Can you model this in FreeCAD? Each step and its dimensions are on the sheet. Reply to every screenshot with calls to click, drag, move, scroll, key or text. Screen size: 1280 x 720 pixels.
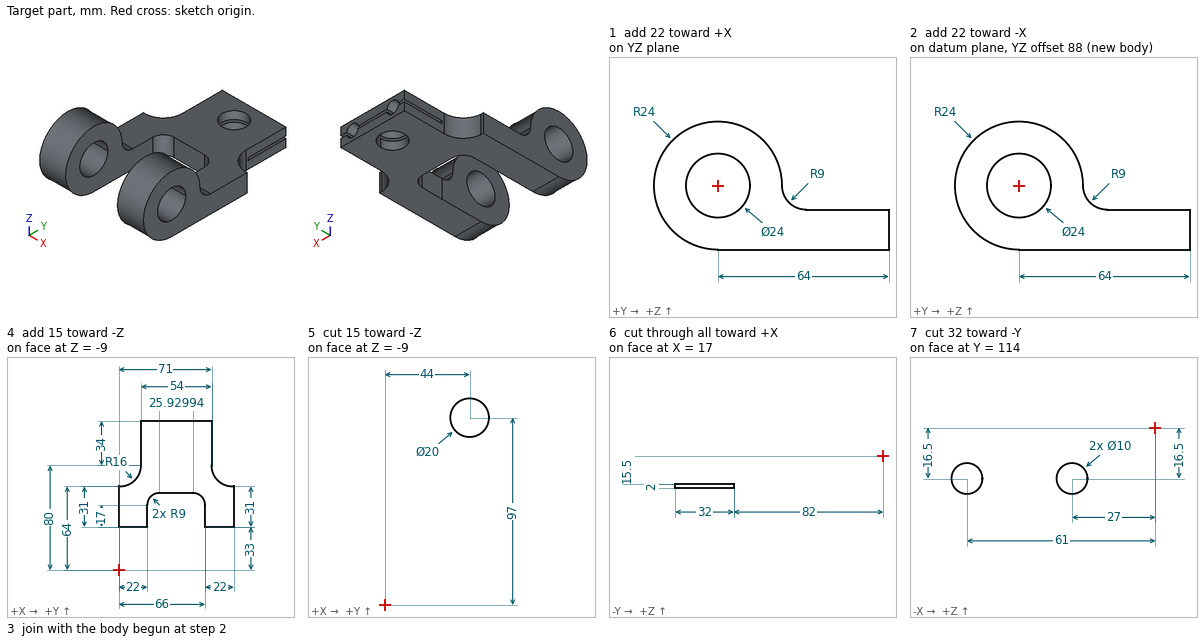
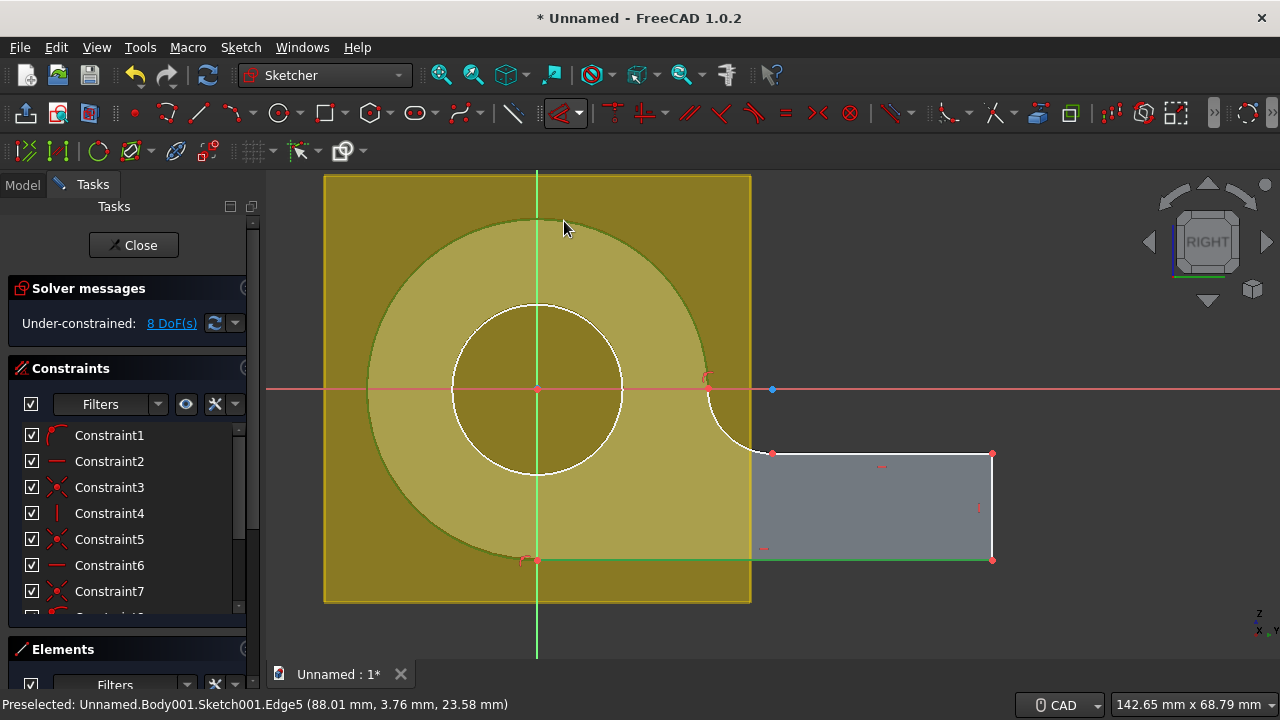
click(754, 114)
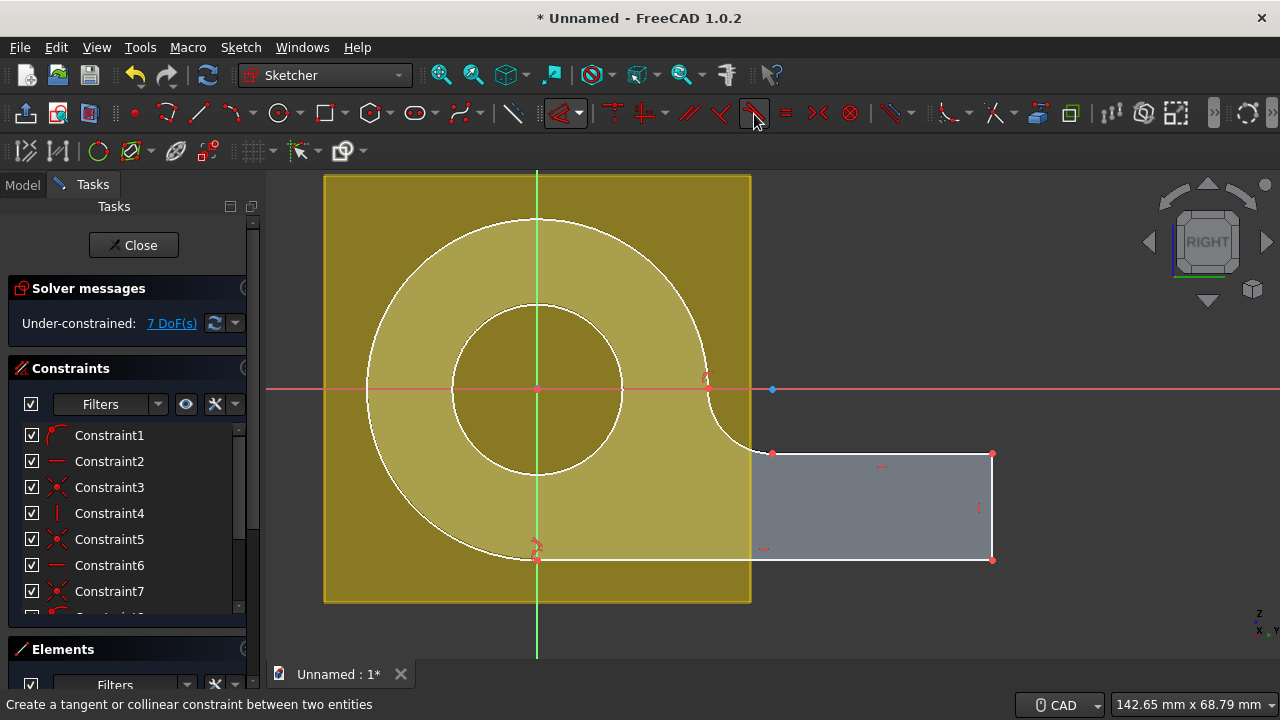
click(926, 454)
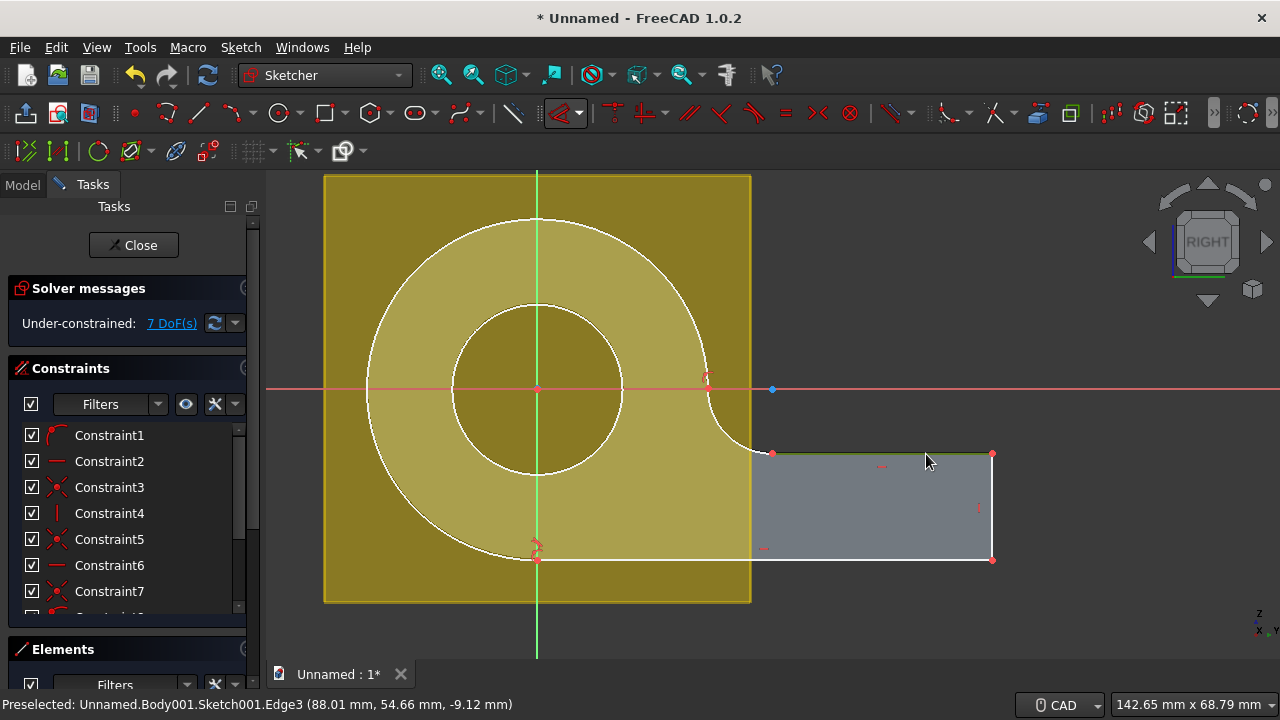
click(715, 418)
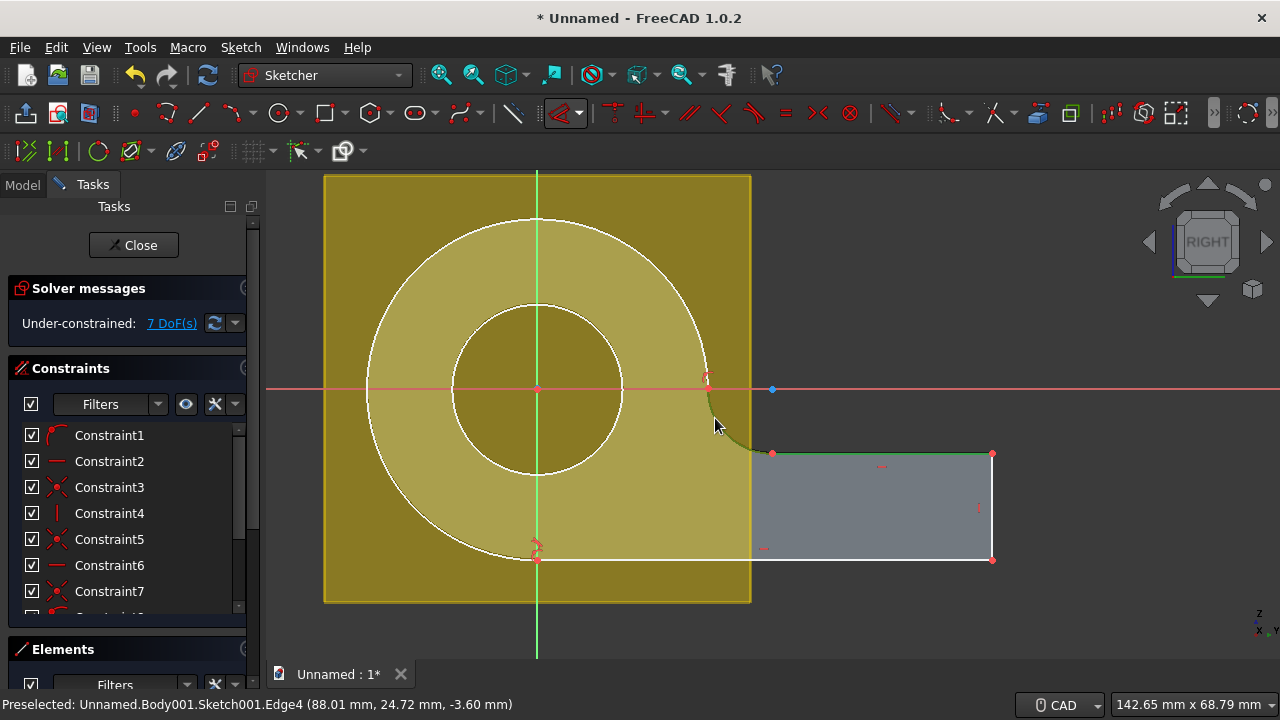
click(754, 114)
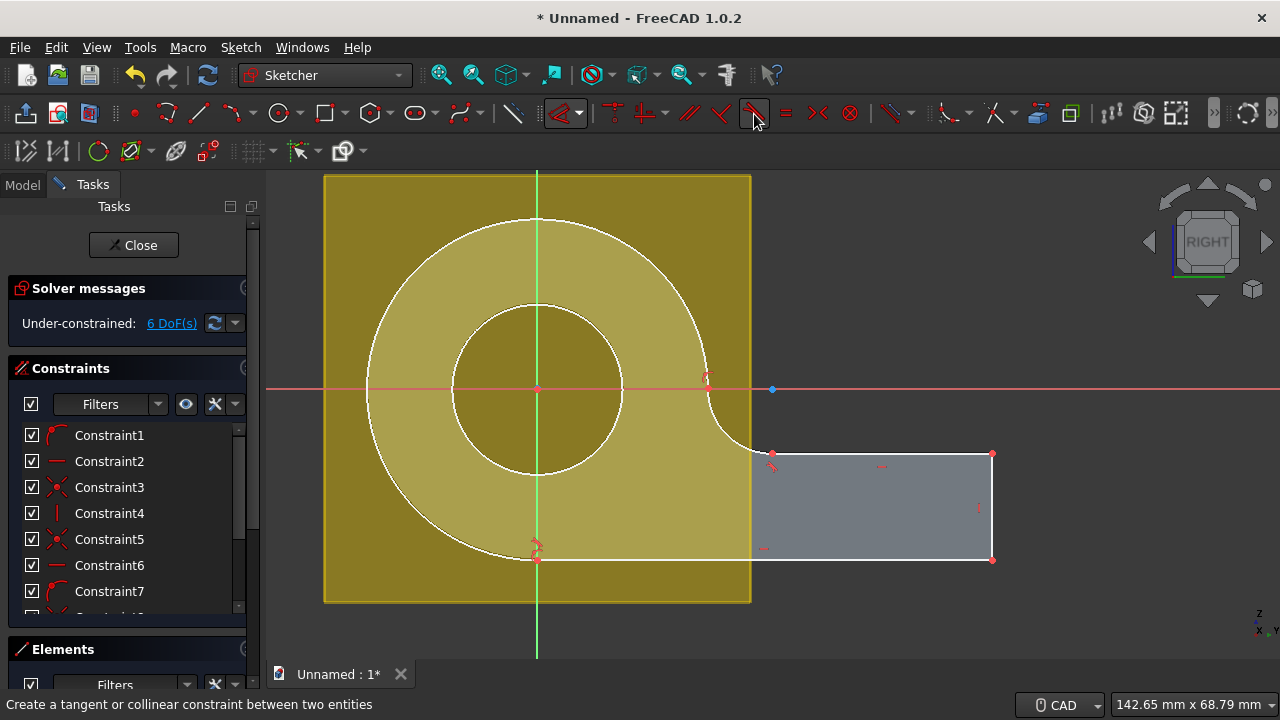
click(715, 418)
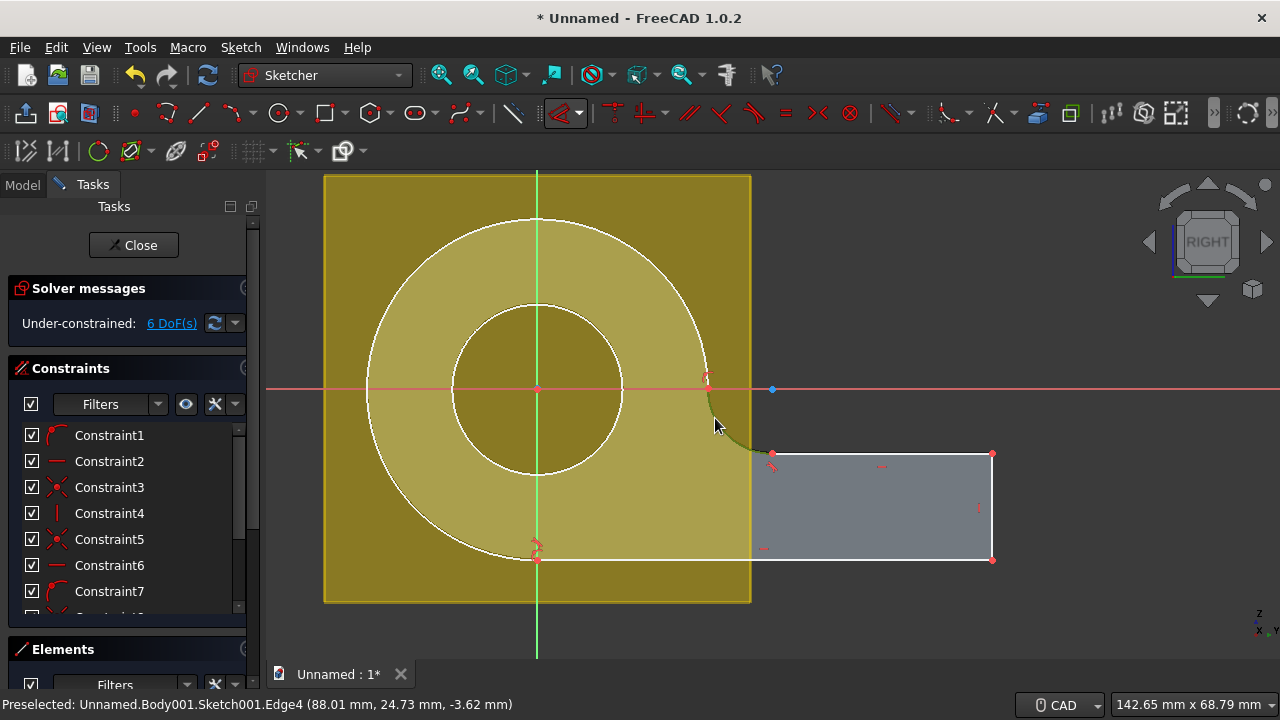
click(564, 221)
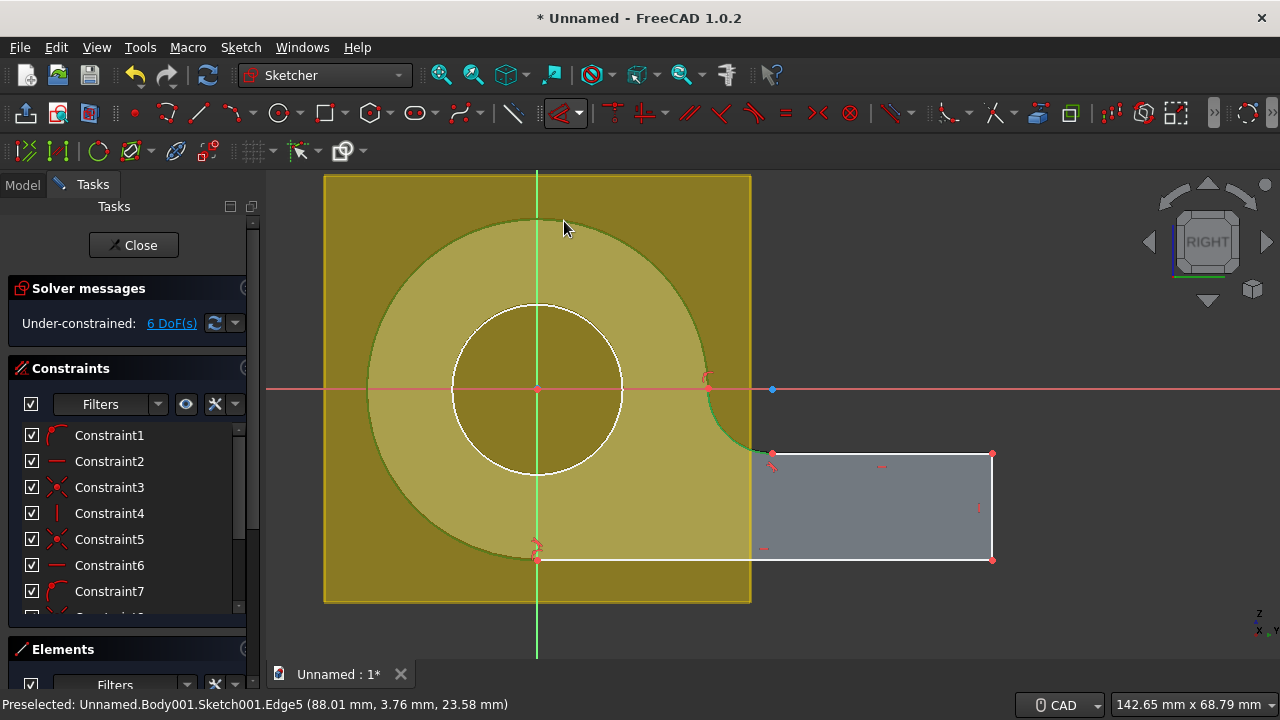
click(754, 114)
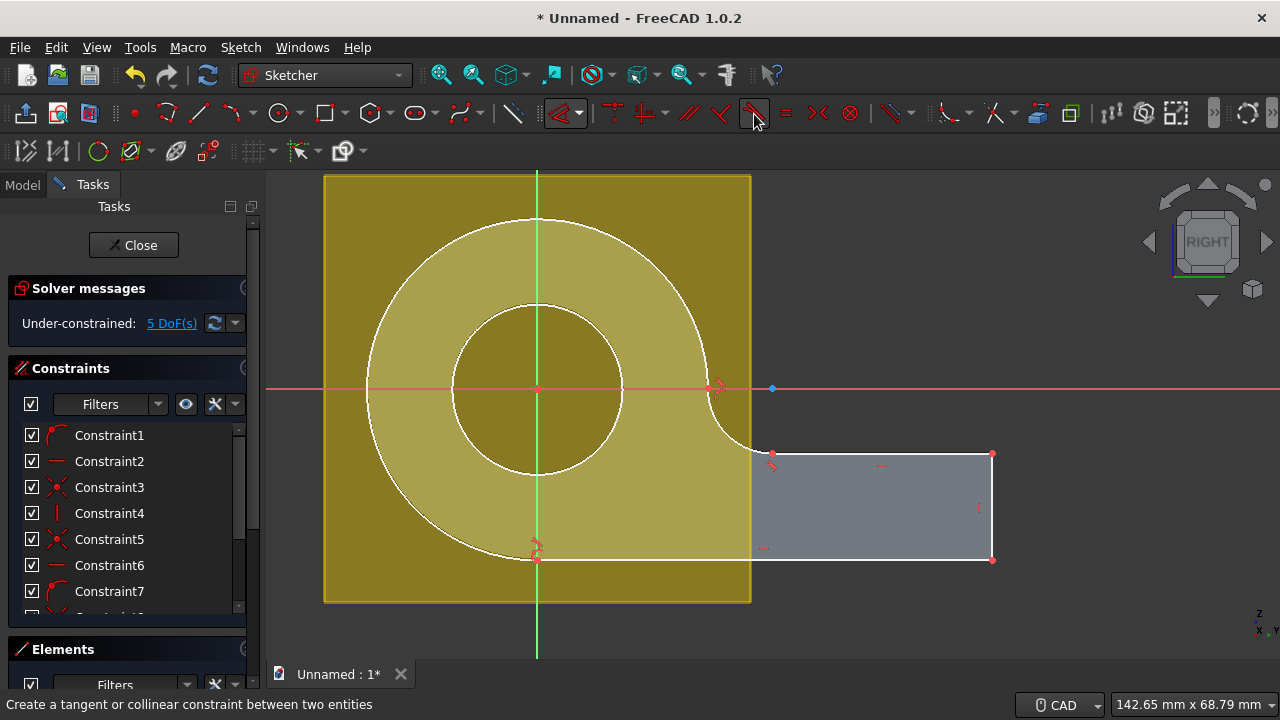
click(773, 389)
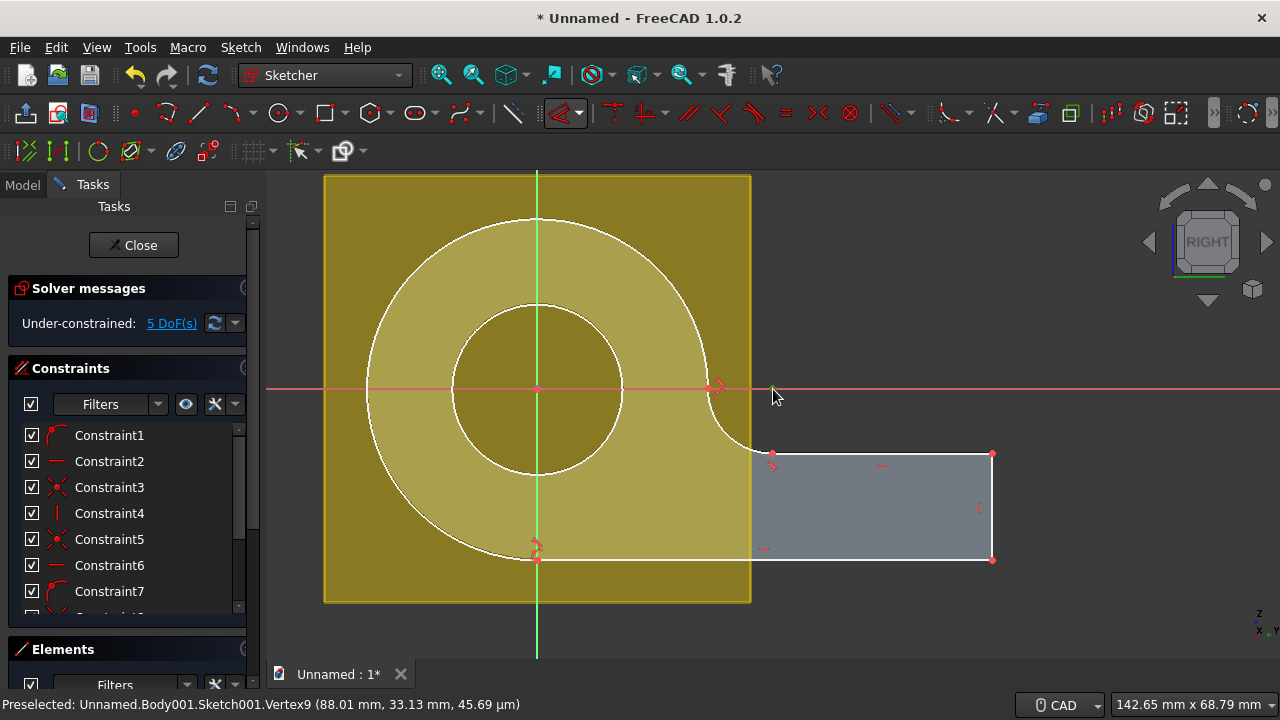
click(411, 389)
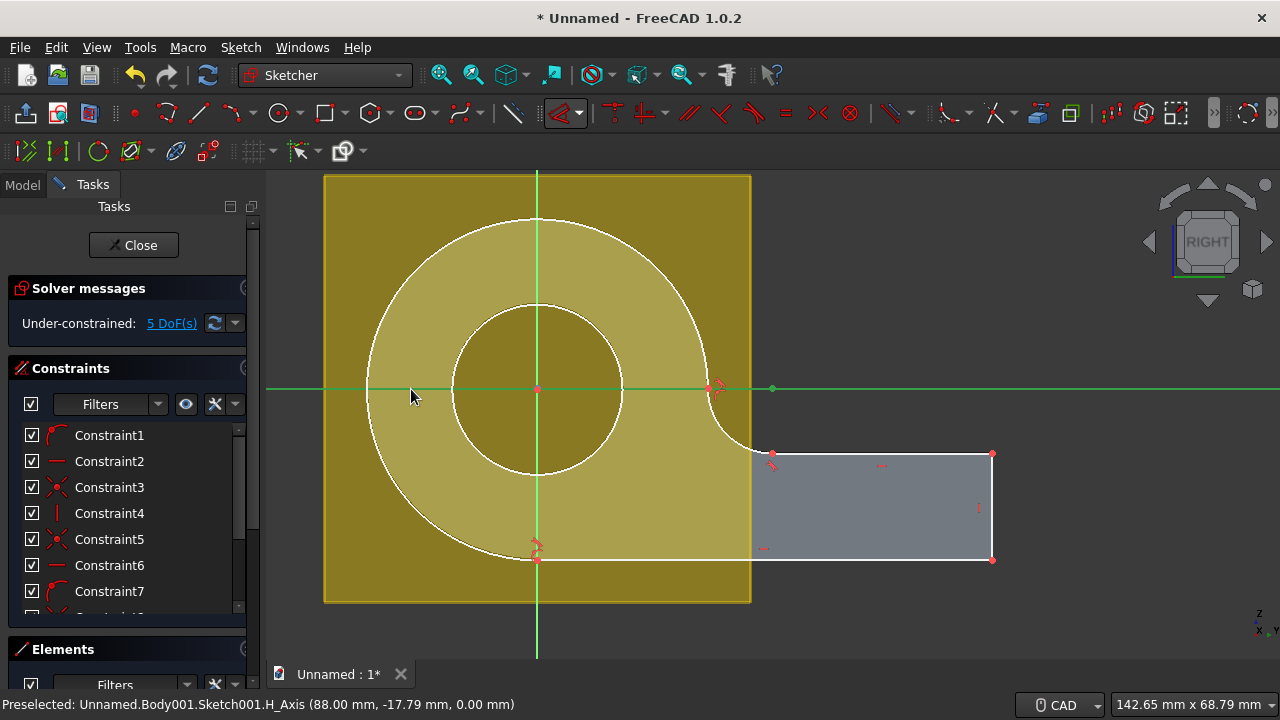
click(614, 114)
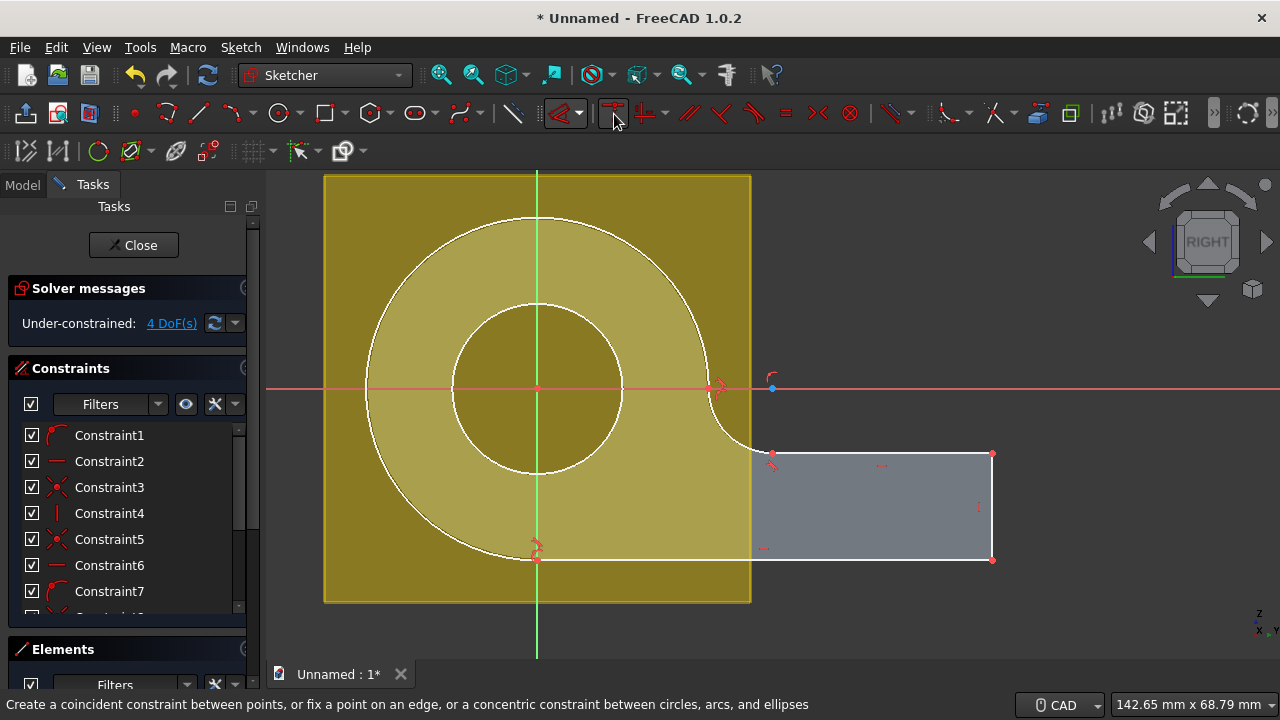
click(716, 418)